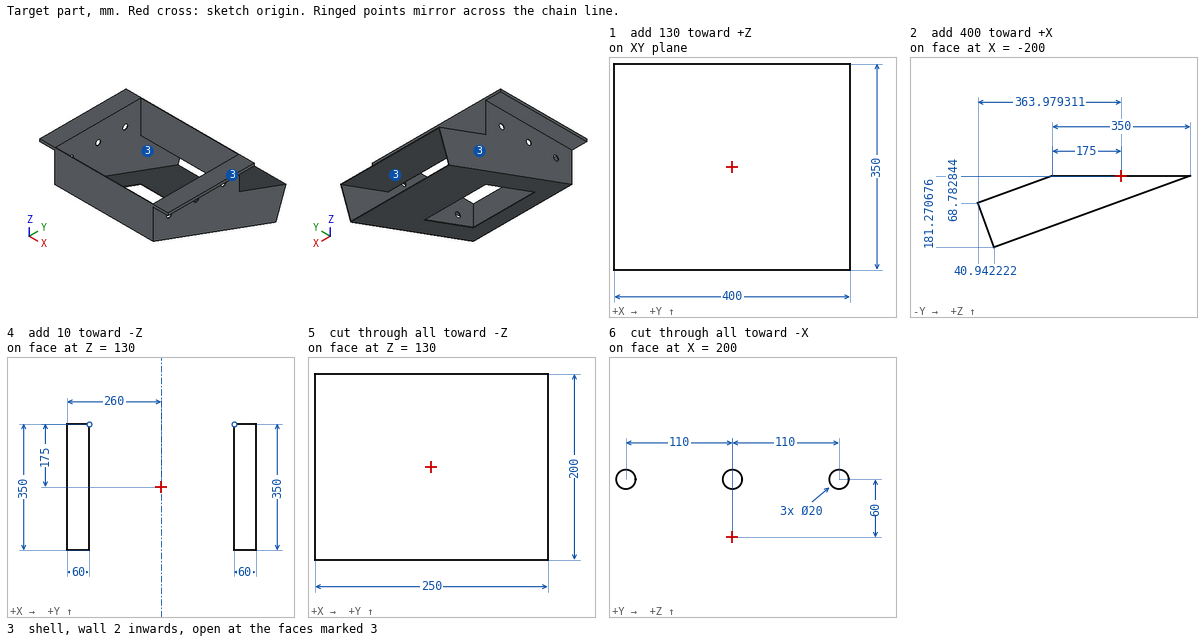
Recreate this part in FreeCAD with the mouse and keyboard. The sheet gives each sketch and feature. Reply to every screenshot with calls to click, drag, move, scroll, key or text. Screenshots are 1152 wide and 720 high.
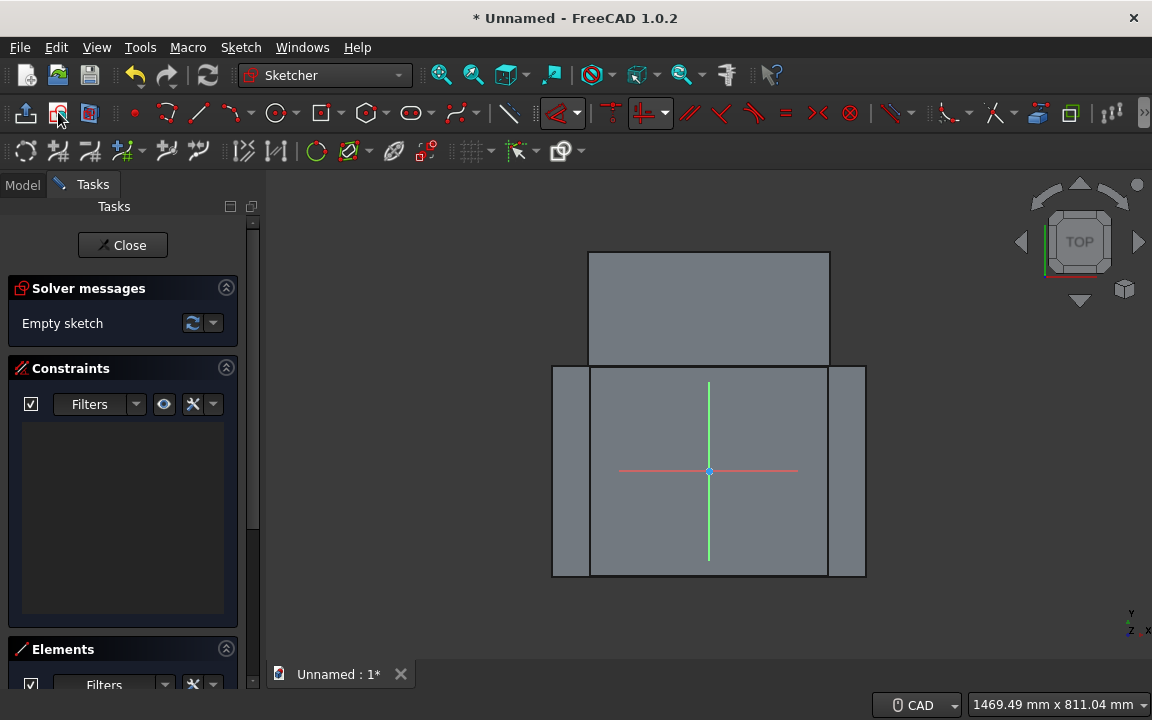
scroll(749, 505, up, 5)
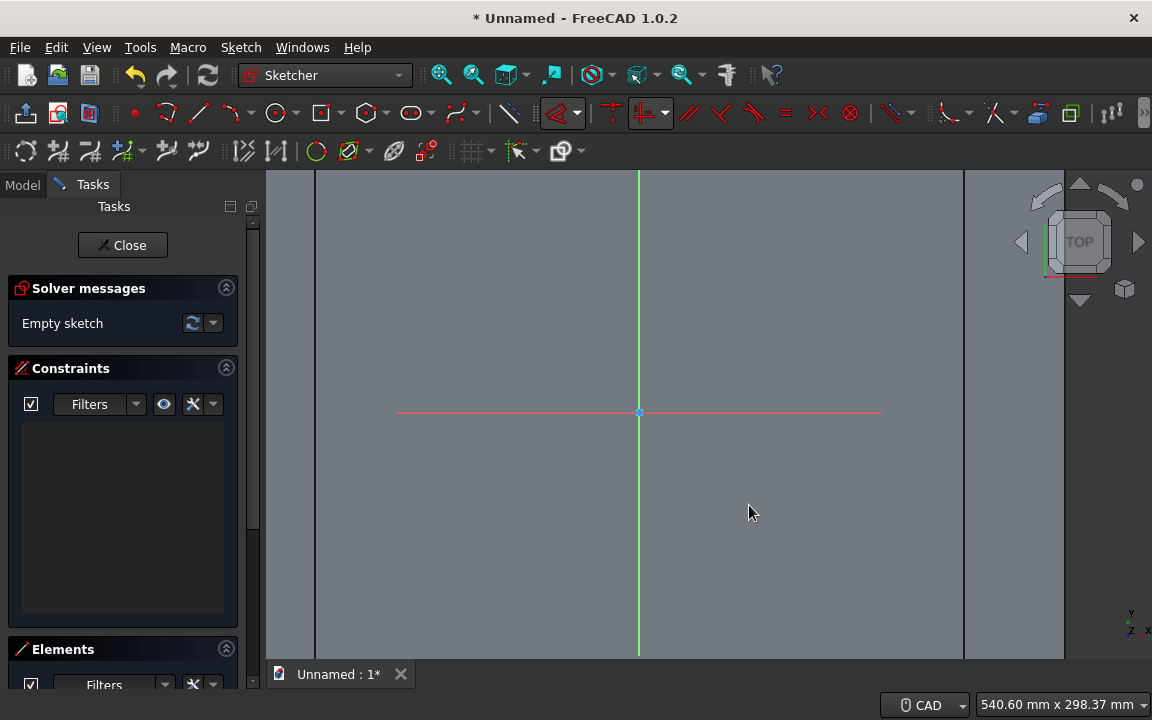
click(322, 114)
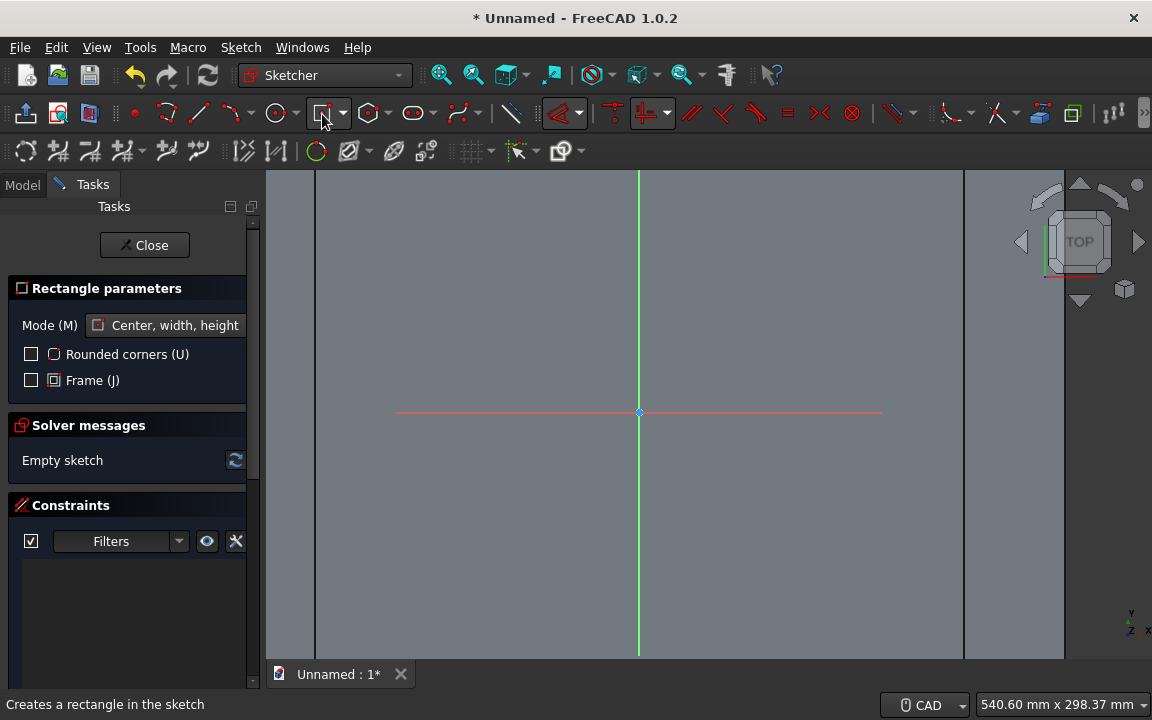
click(639, 413)
move(844, 249)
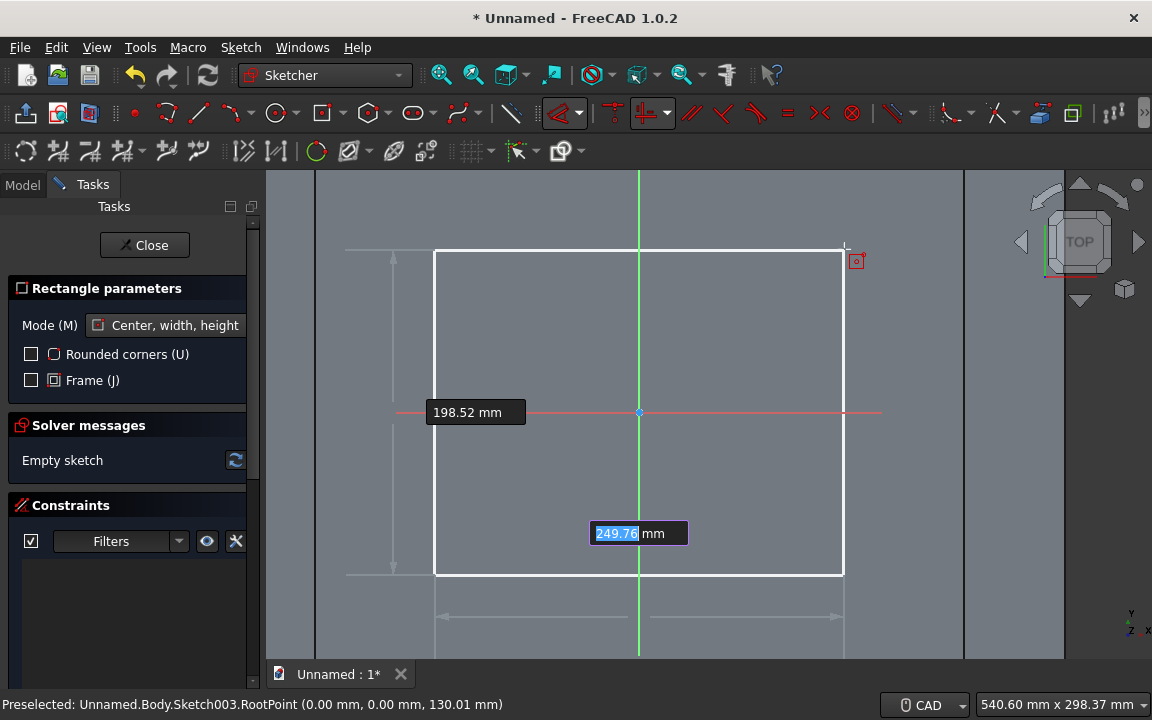
text(250)
key(Tab)
text(200)
key(Return)
key(Escape)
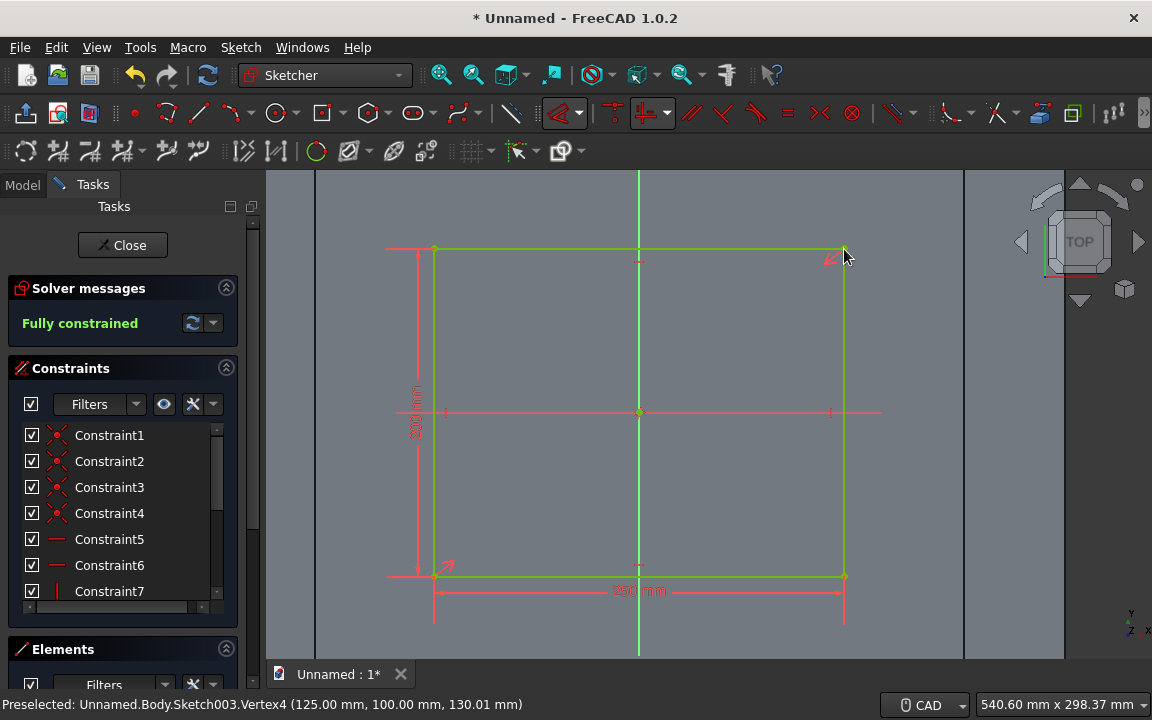
click(123, 245)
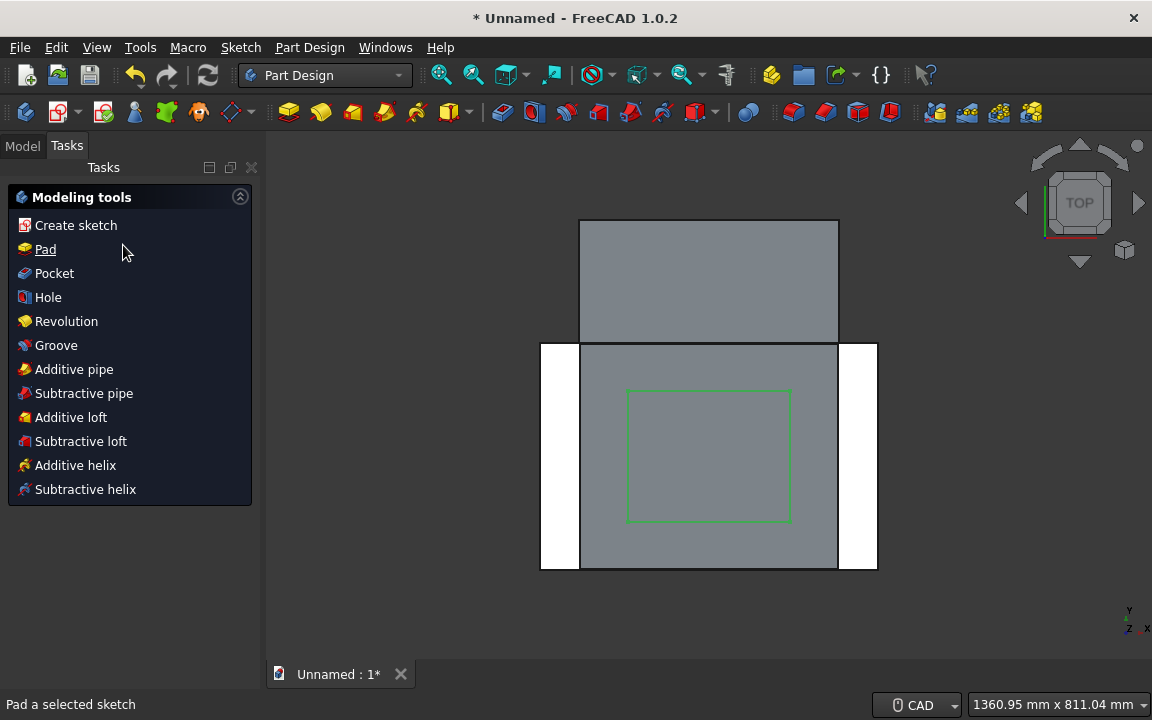
click(504, 112)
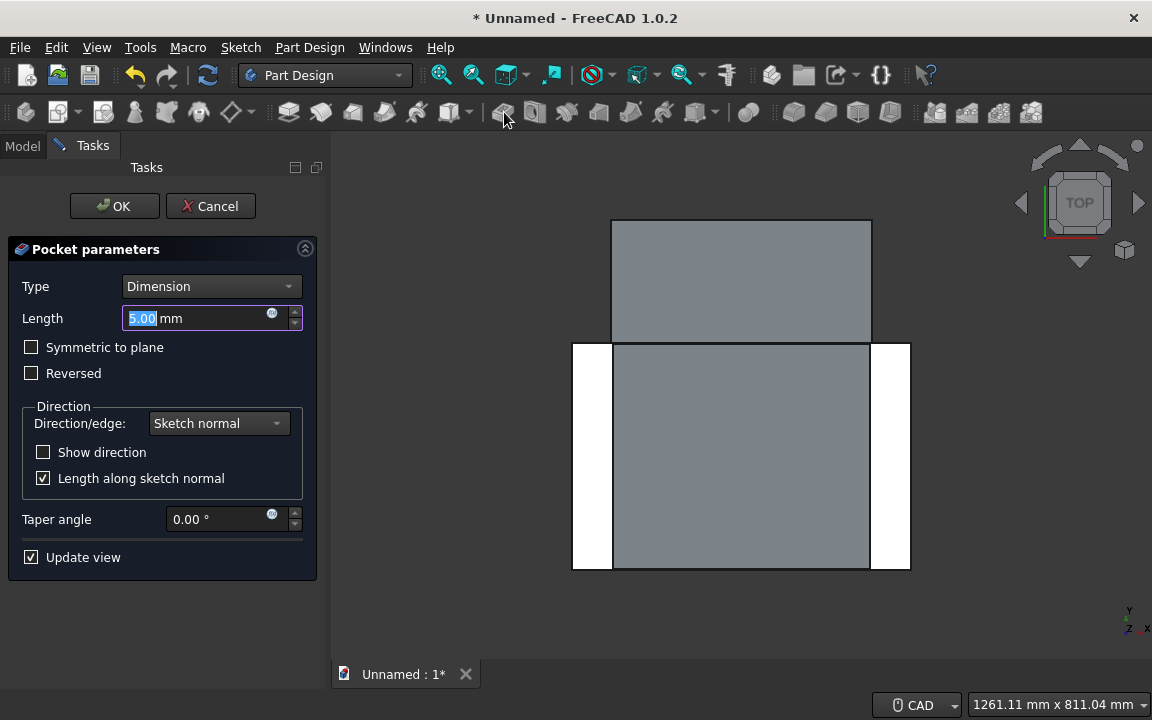
click(212, 286)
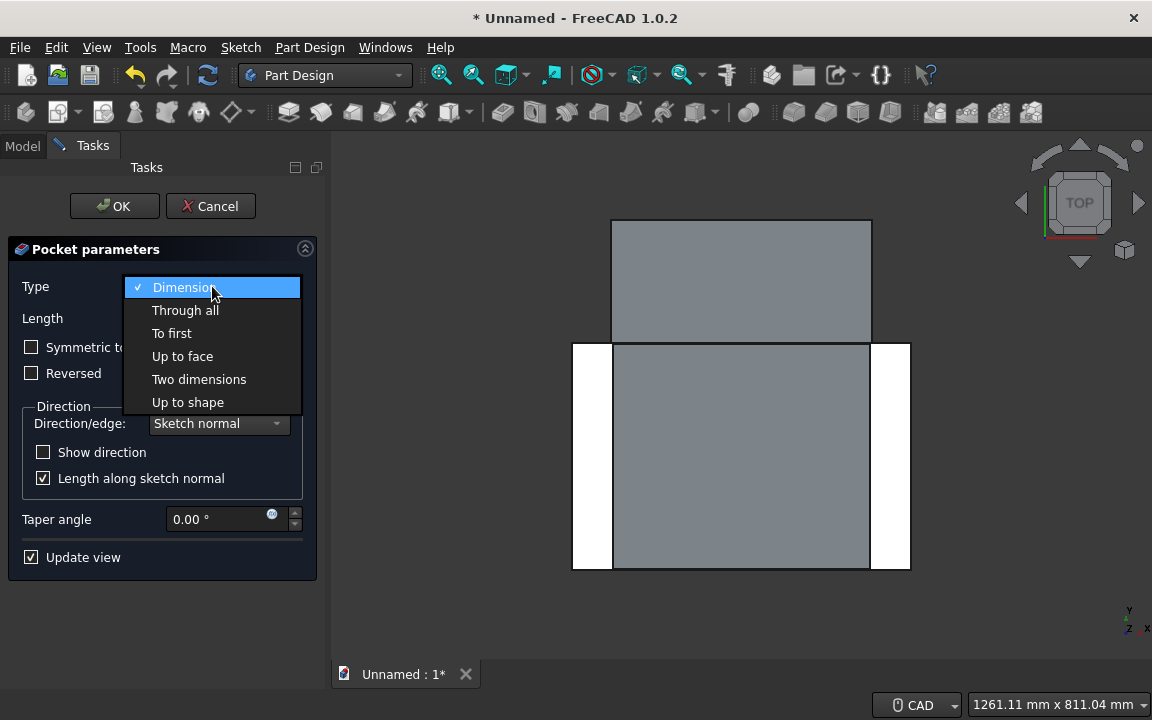
click(212, 310)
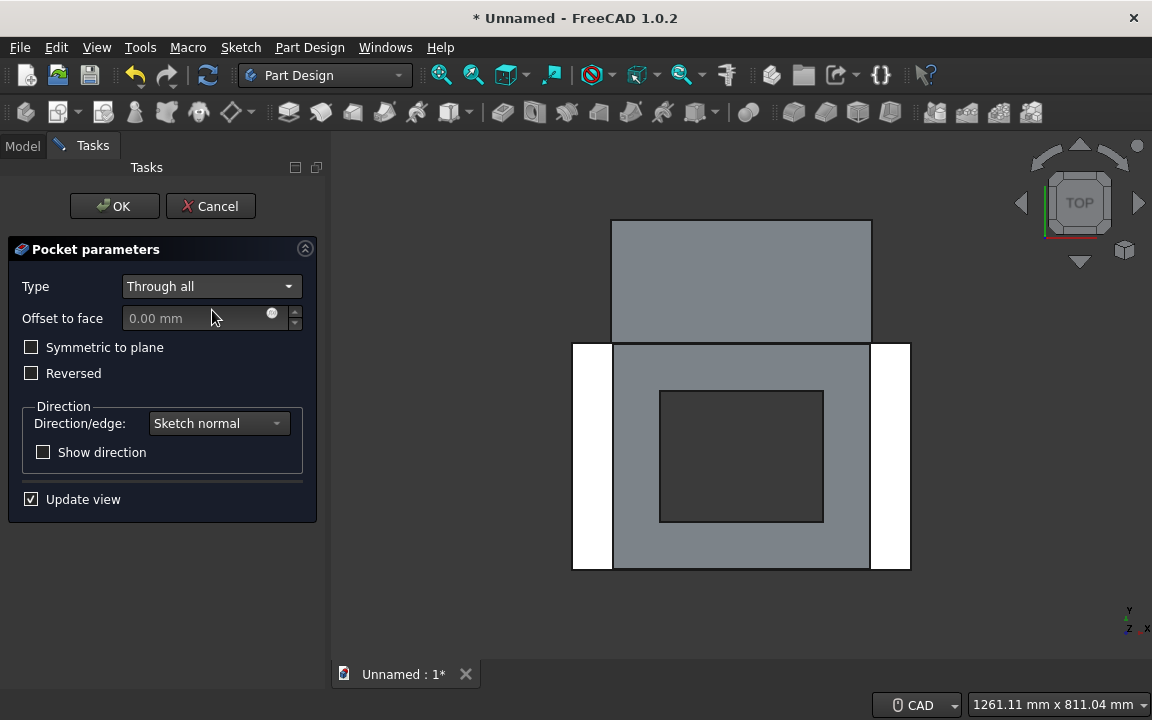
click(115, 206)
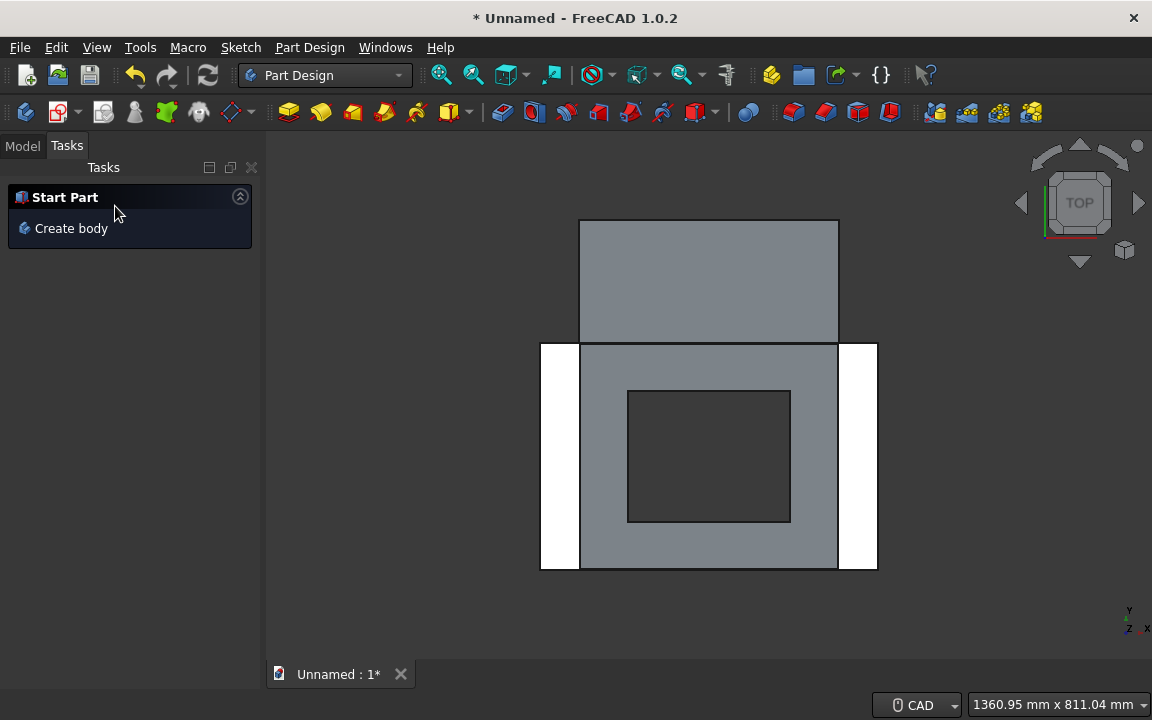
key(0)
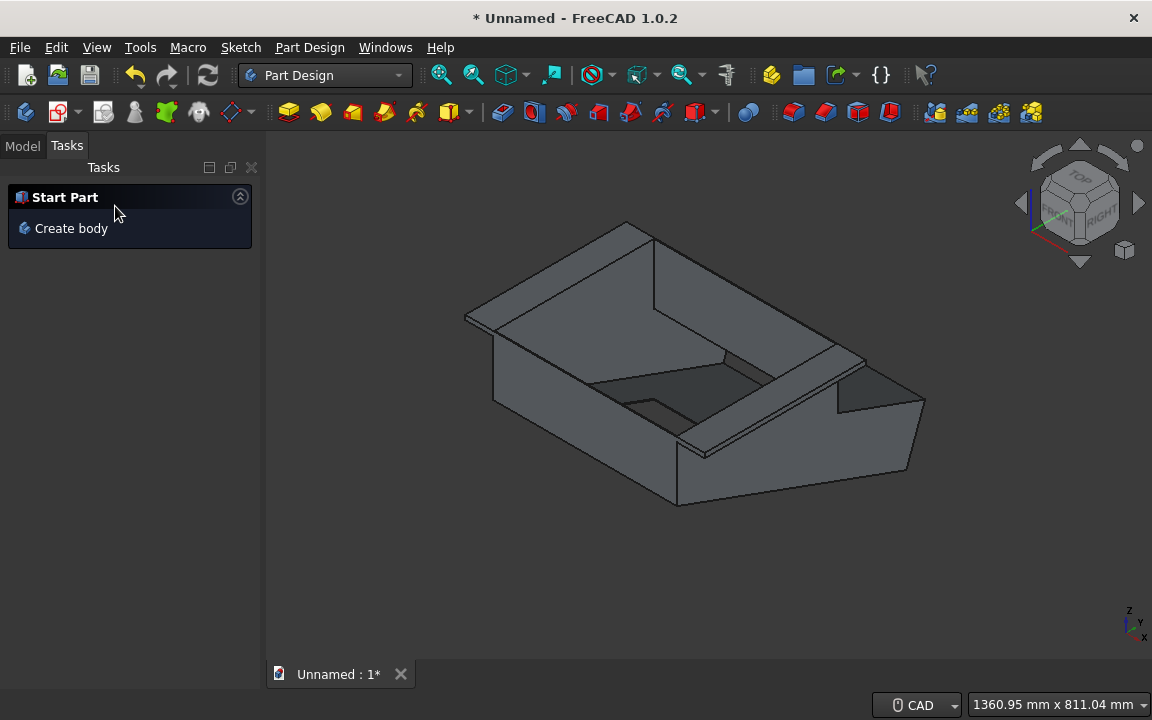
click(801, 427)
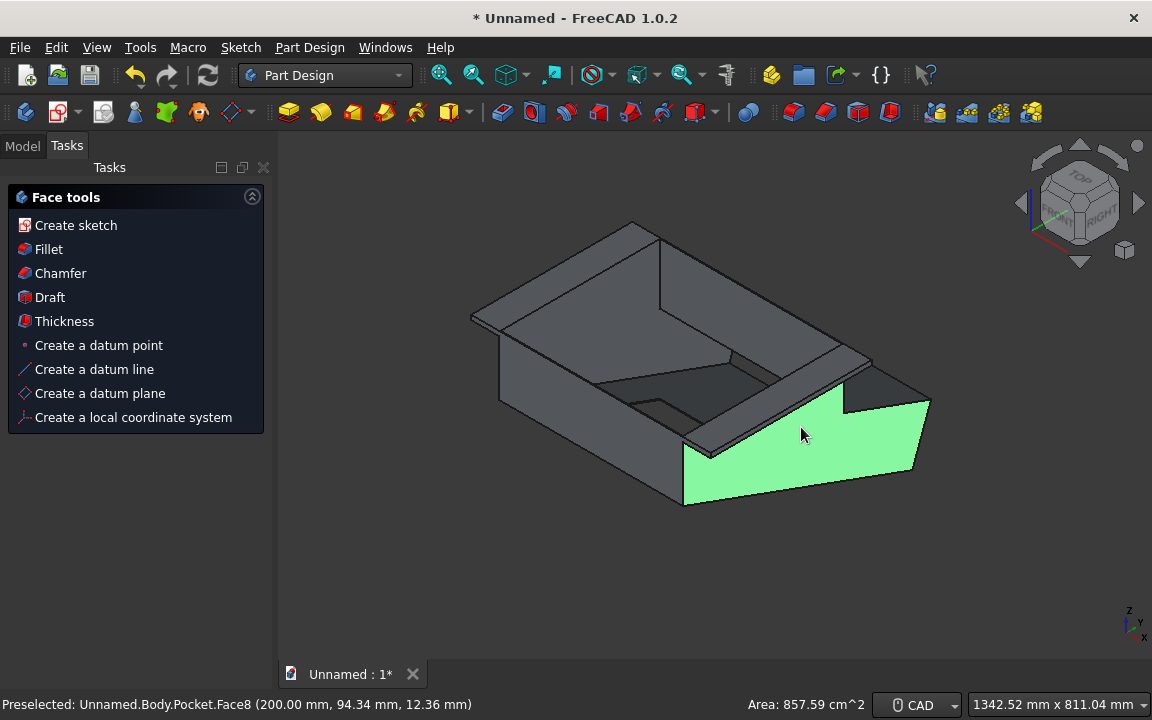
click(58, 112)